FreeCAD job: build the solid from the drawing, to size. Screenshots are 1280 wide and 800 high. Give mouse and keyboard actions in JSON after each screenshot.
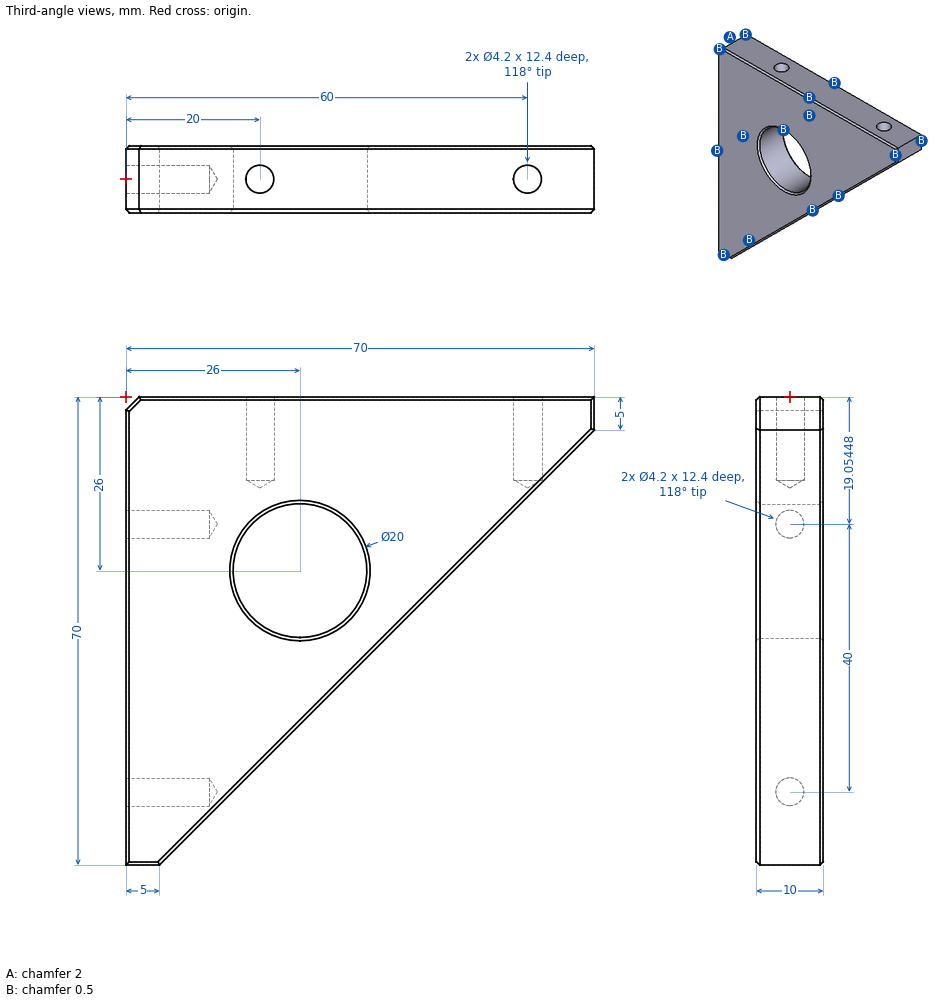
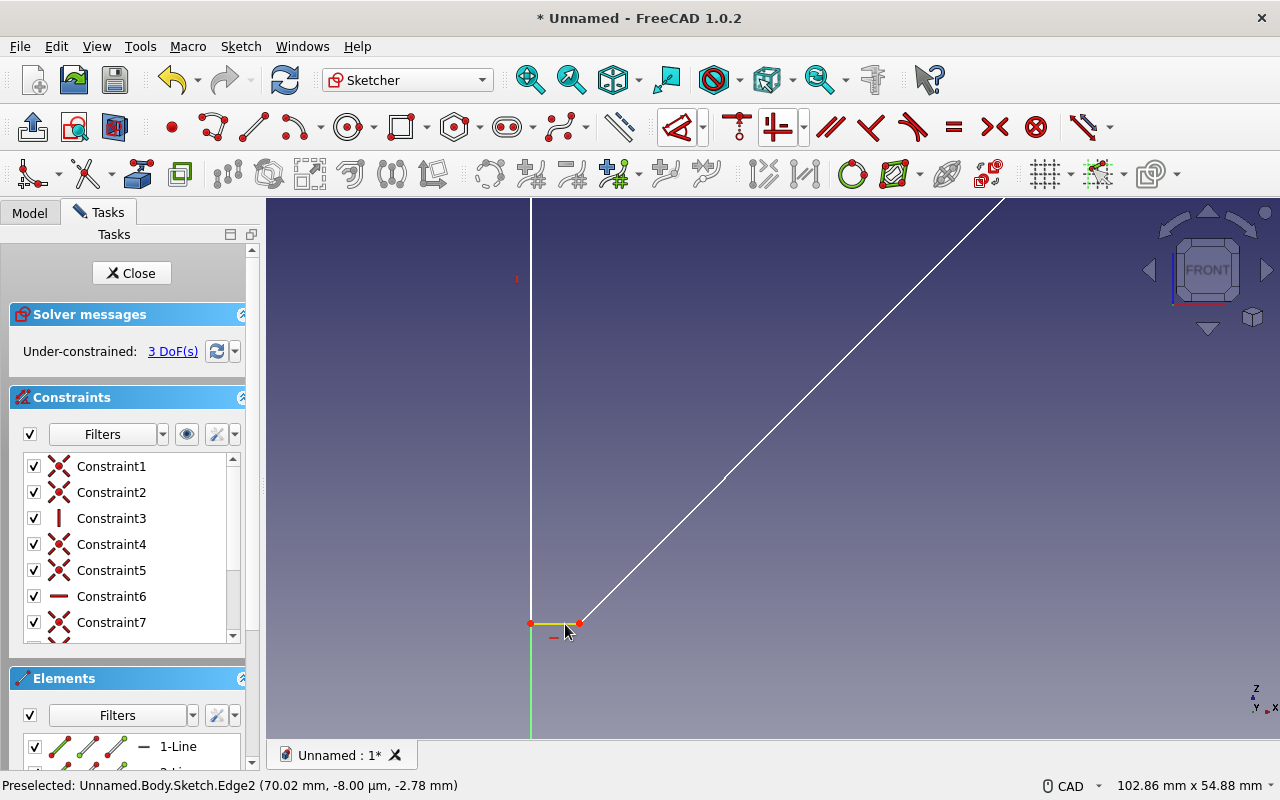
{"action": "left_click", "coordinate": [565, 624]}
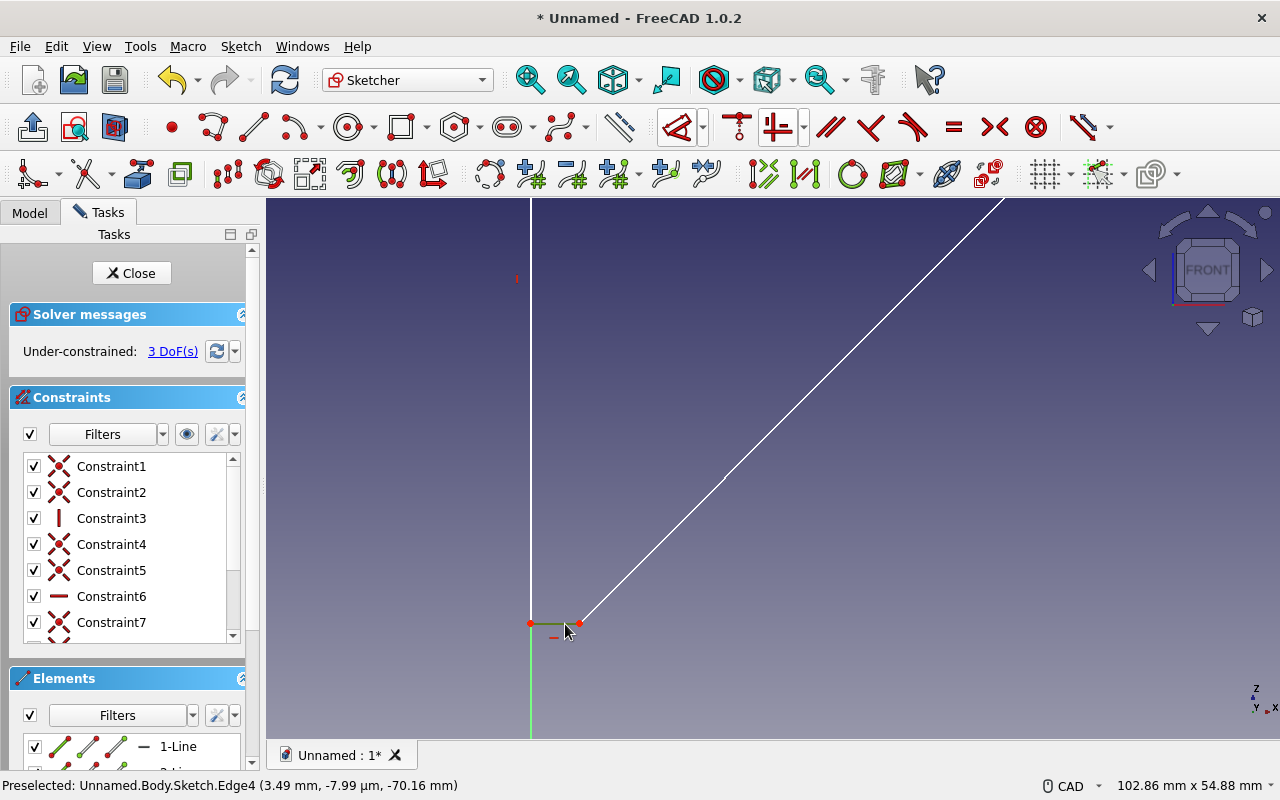
{"action": "key", "text": "l"}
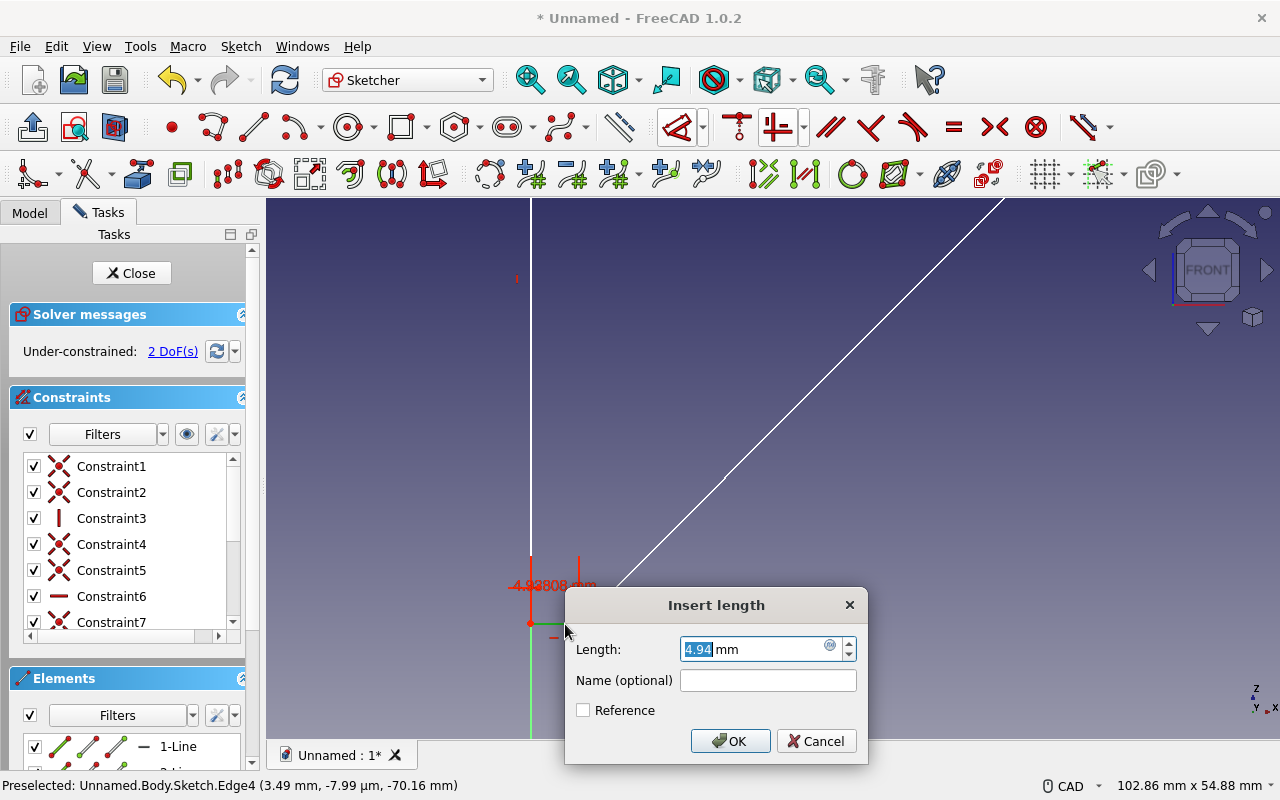
{"action": "type", "text": "5"}
{"action": "key", "text": "Return"}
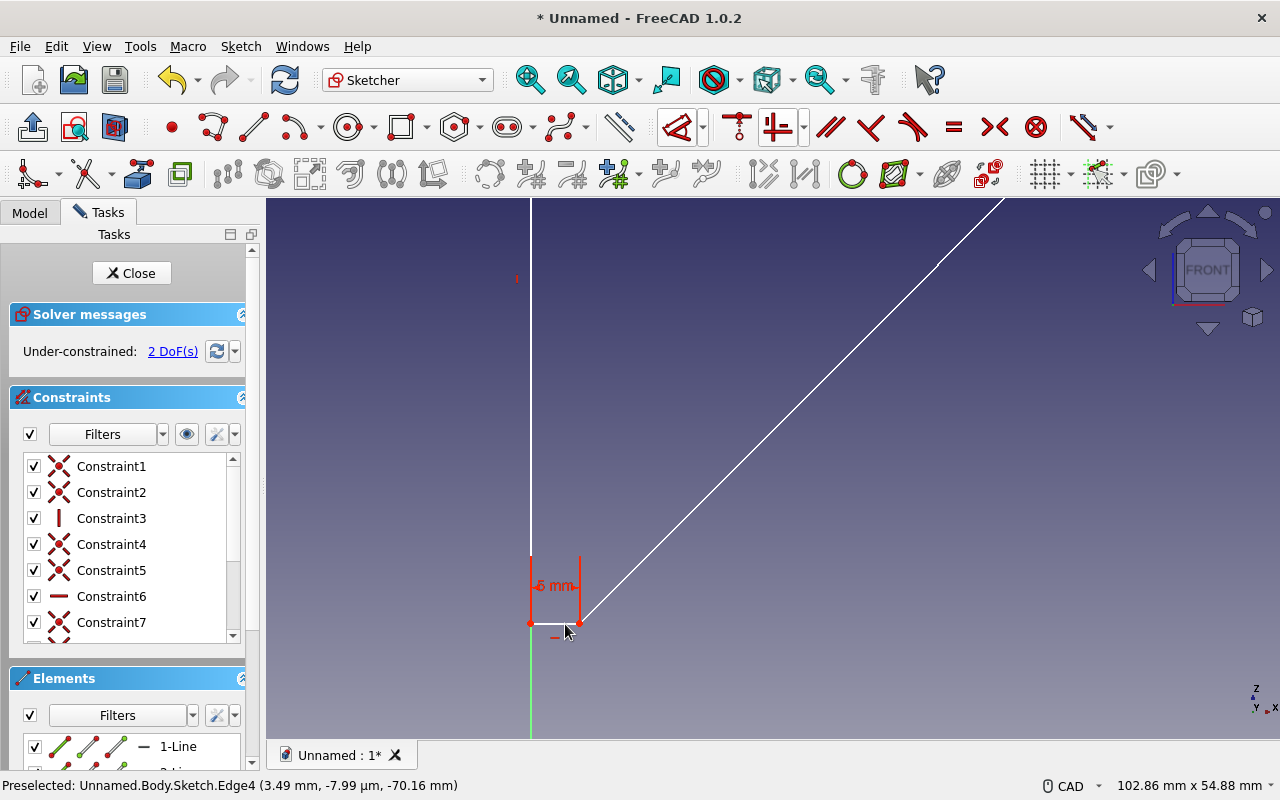
{"action": "scroll", "coordinate": [565, 625], "scroll_direction": "down", "scroll_amount": 4}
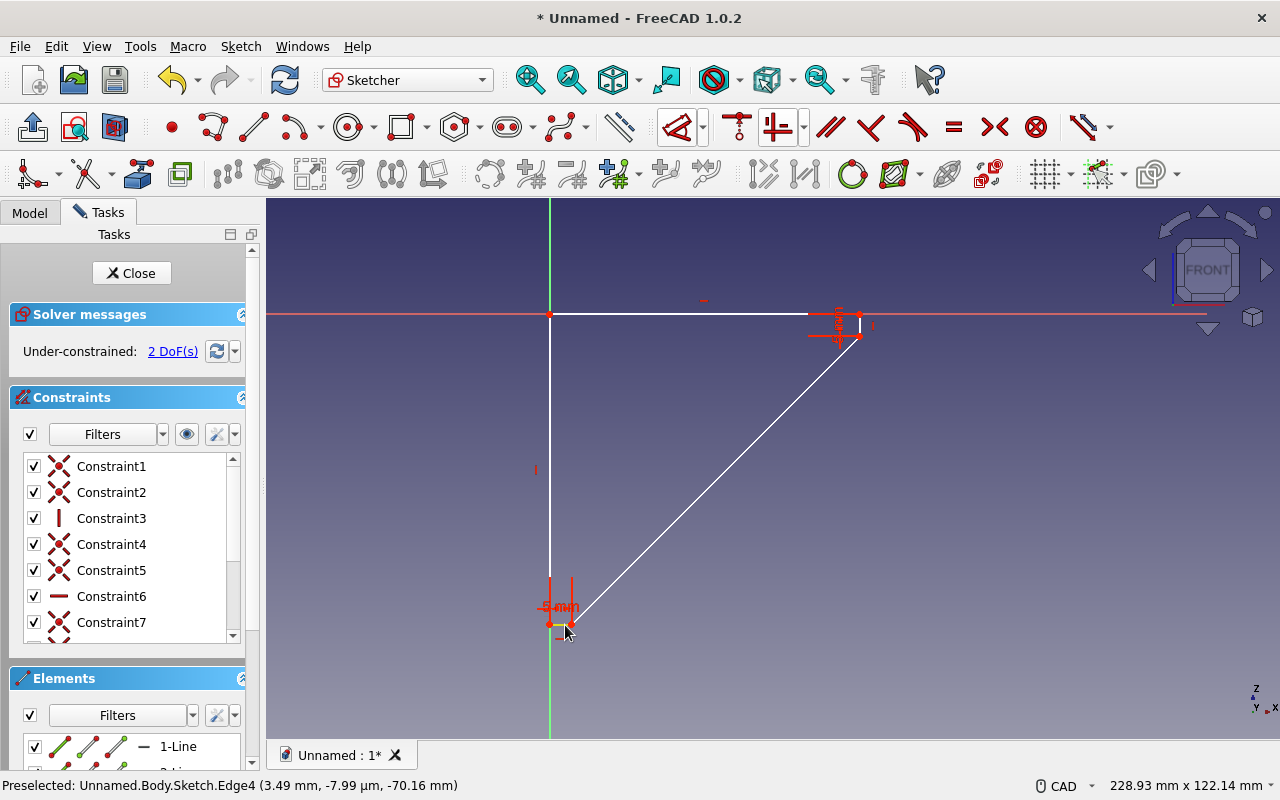
{"action": "left_click", "coordinate": [643, 314]}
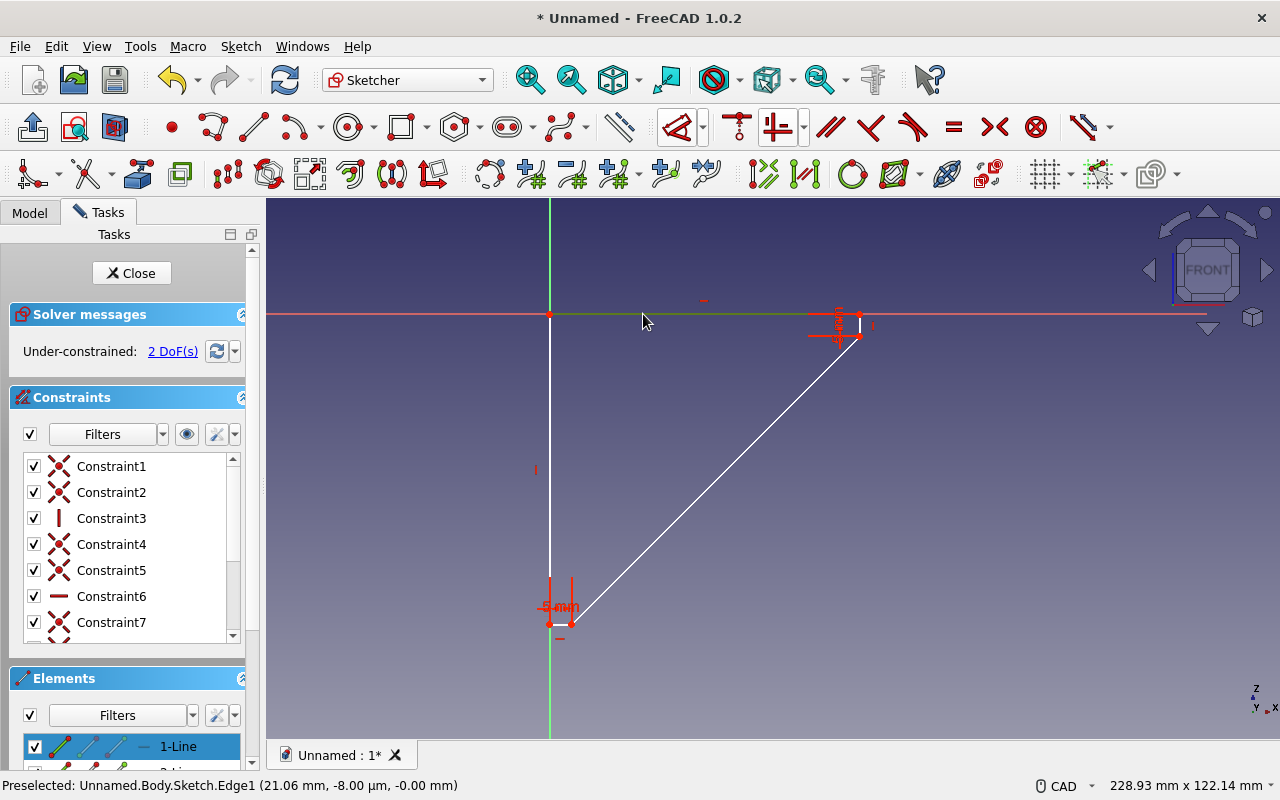
{"action": "key", "text": "l"}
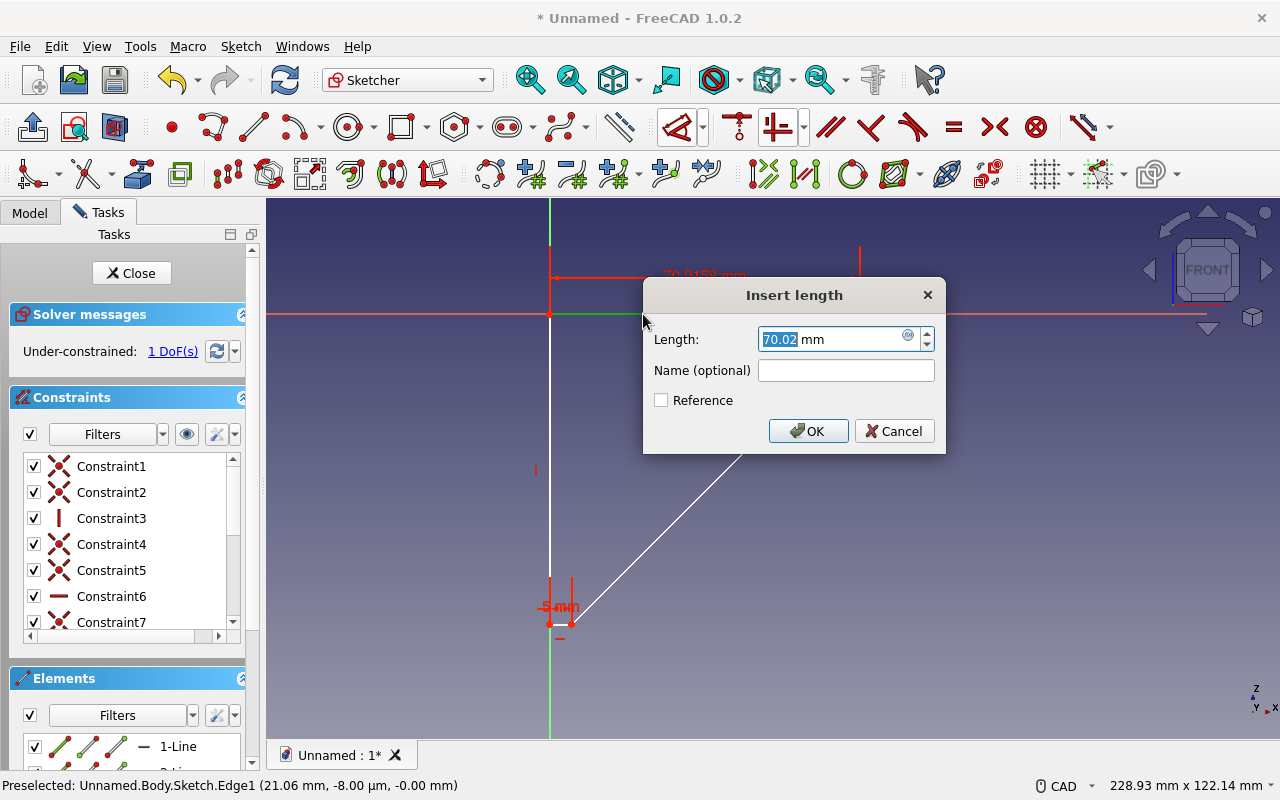
{"action": "type", "text": "70"}
{"action": "key", "text": "Return"}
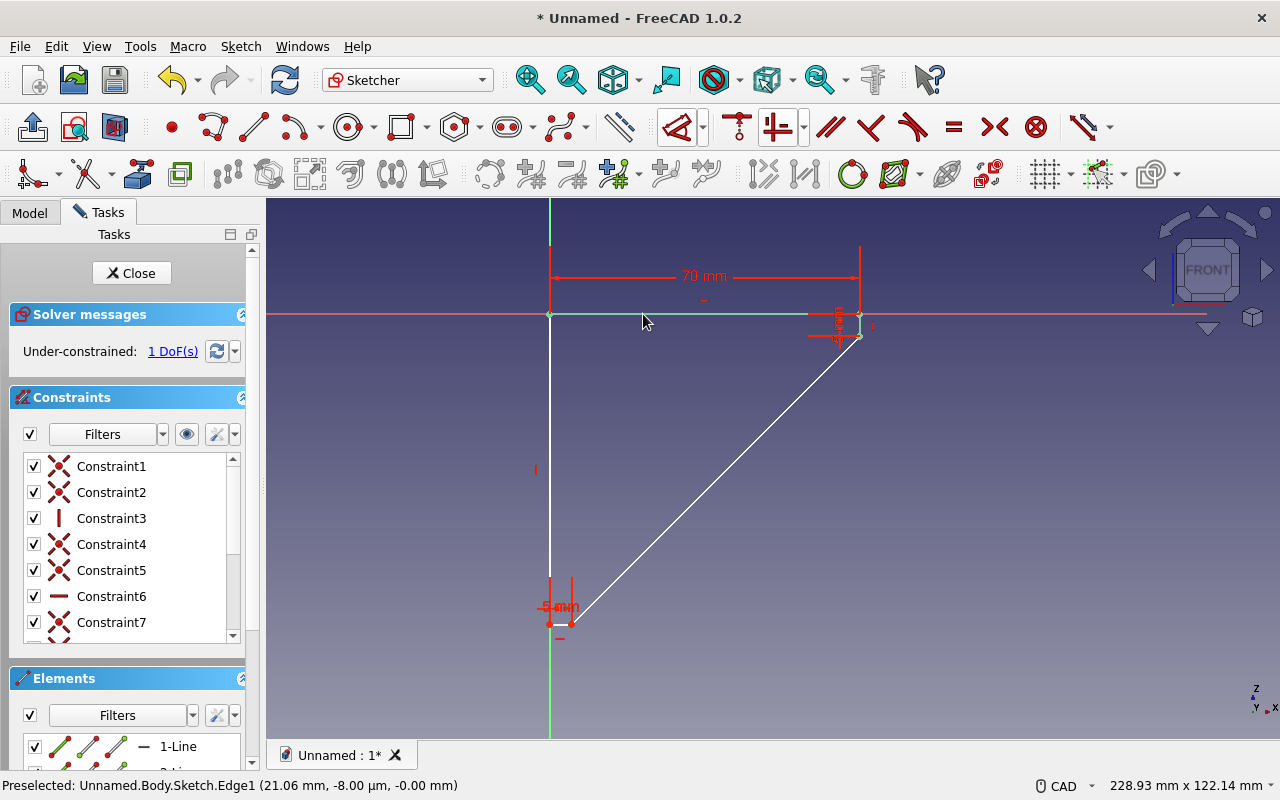
{"action": "left_click", "coordinate": [550, 532]}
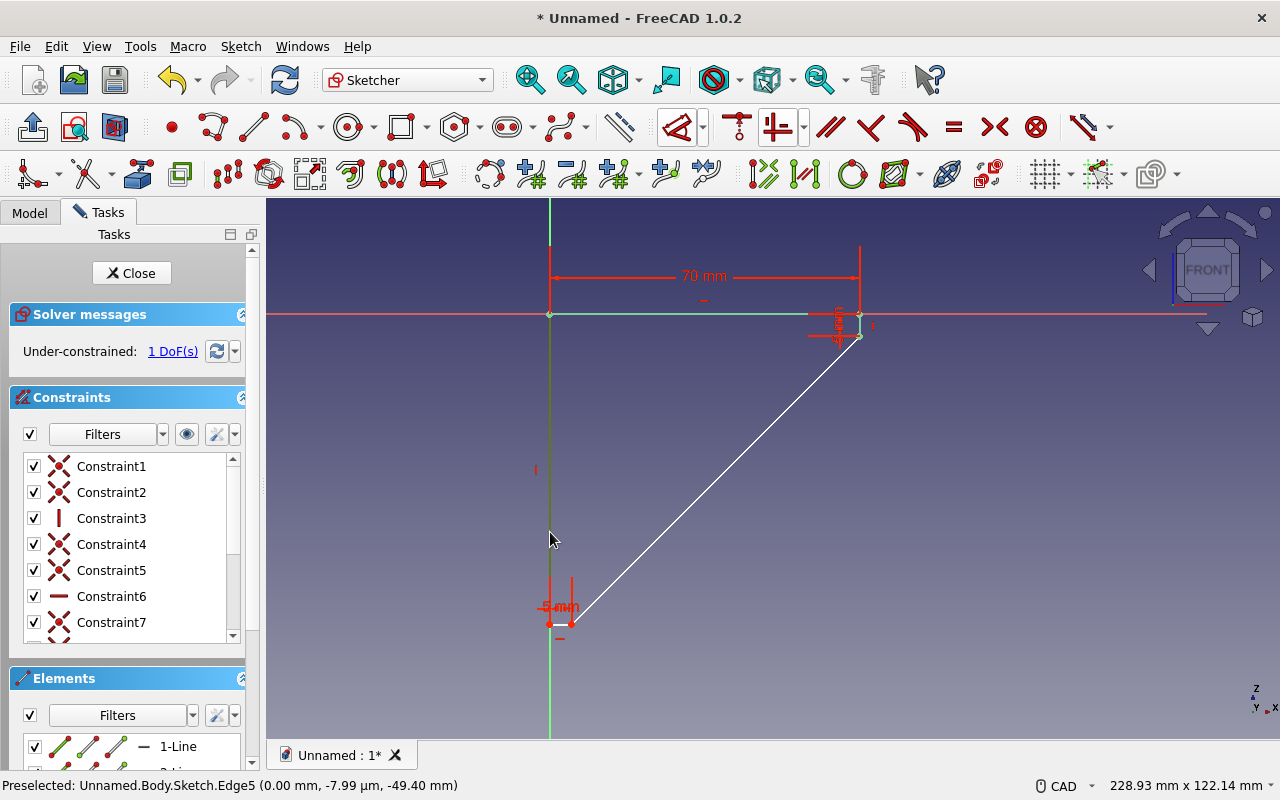
{"action": "left_click", "coordinate": [702, 128]}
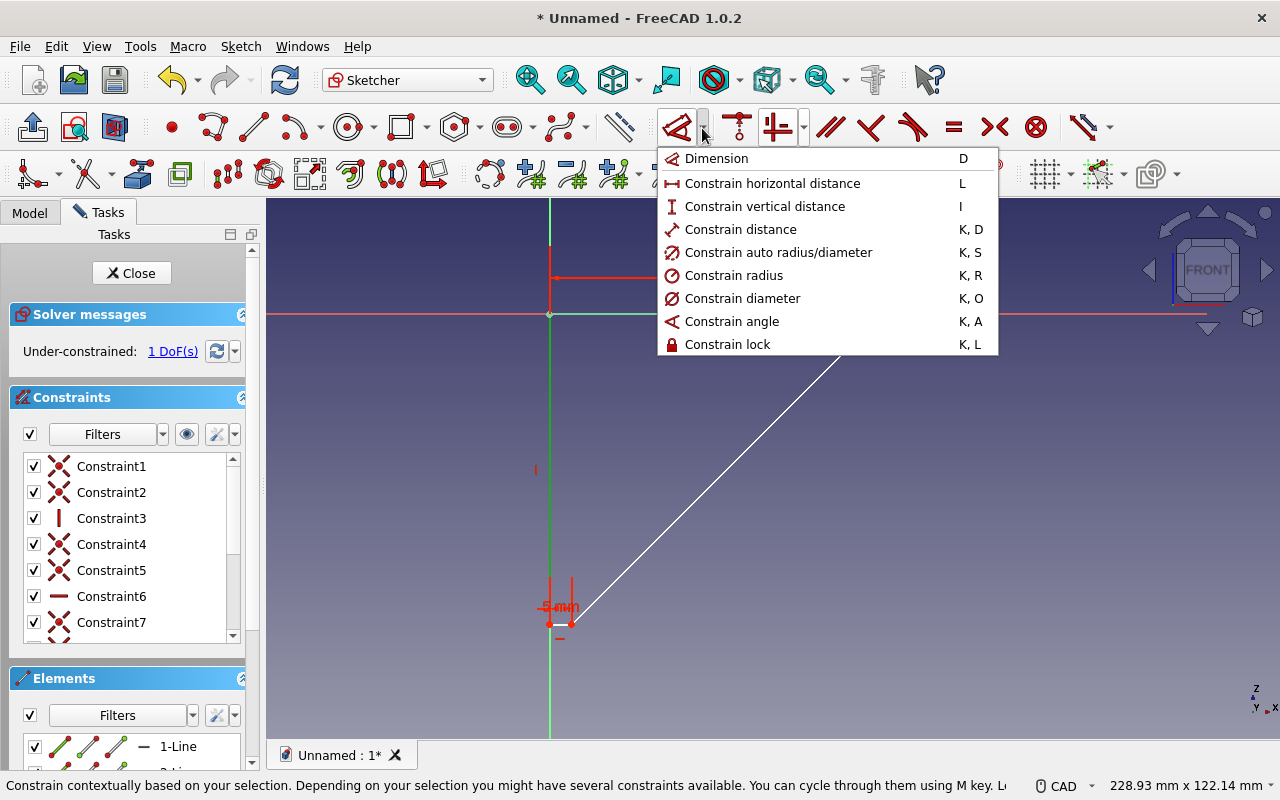
{"action": "left_click", "coordinate": [828, 206]}